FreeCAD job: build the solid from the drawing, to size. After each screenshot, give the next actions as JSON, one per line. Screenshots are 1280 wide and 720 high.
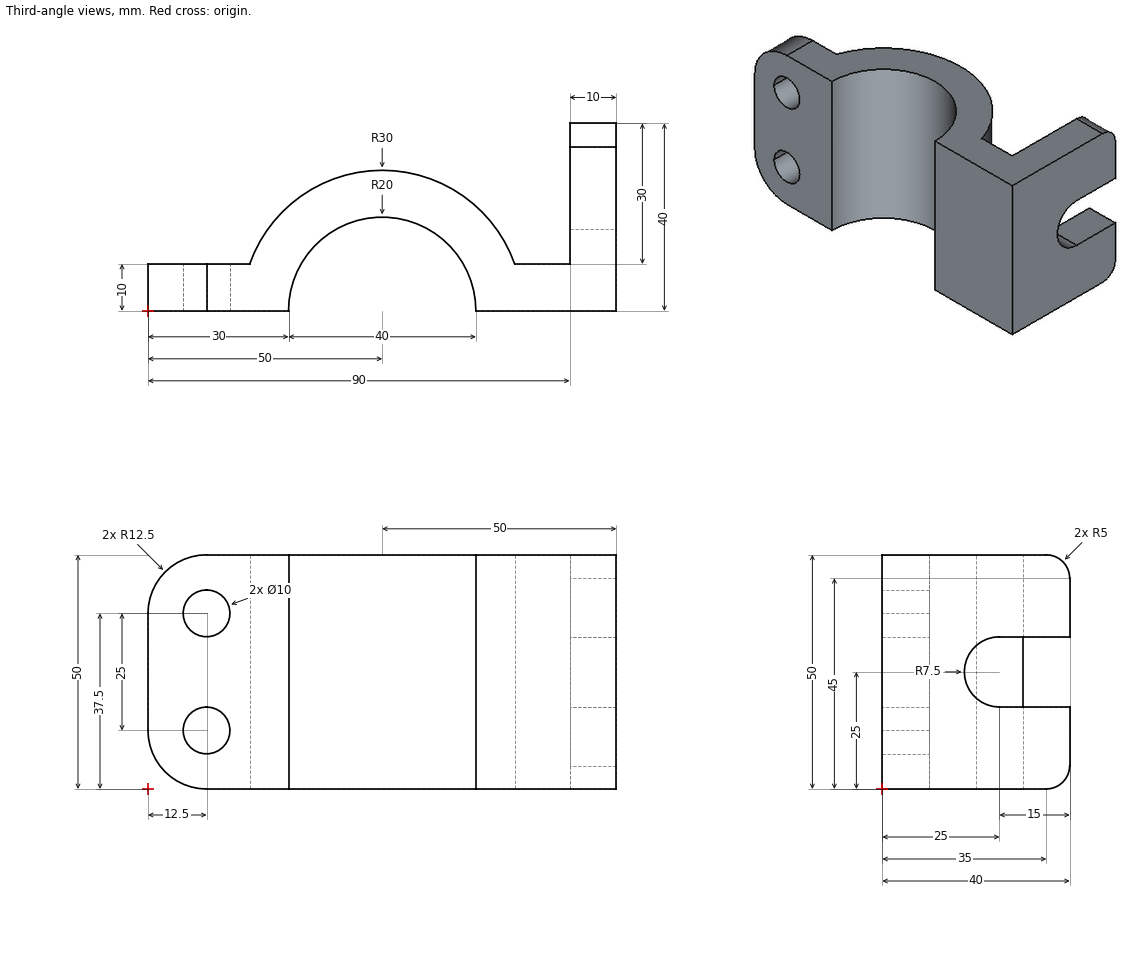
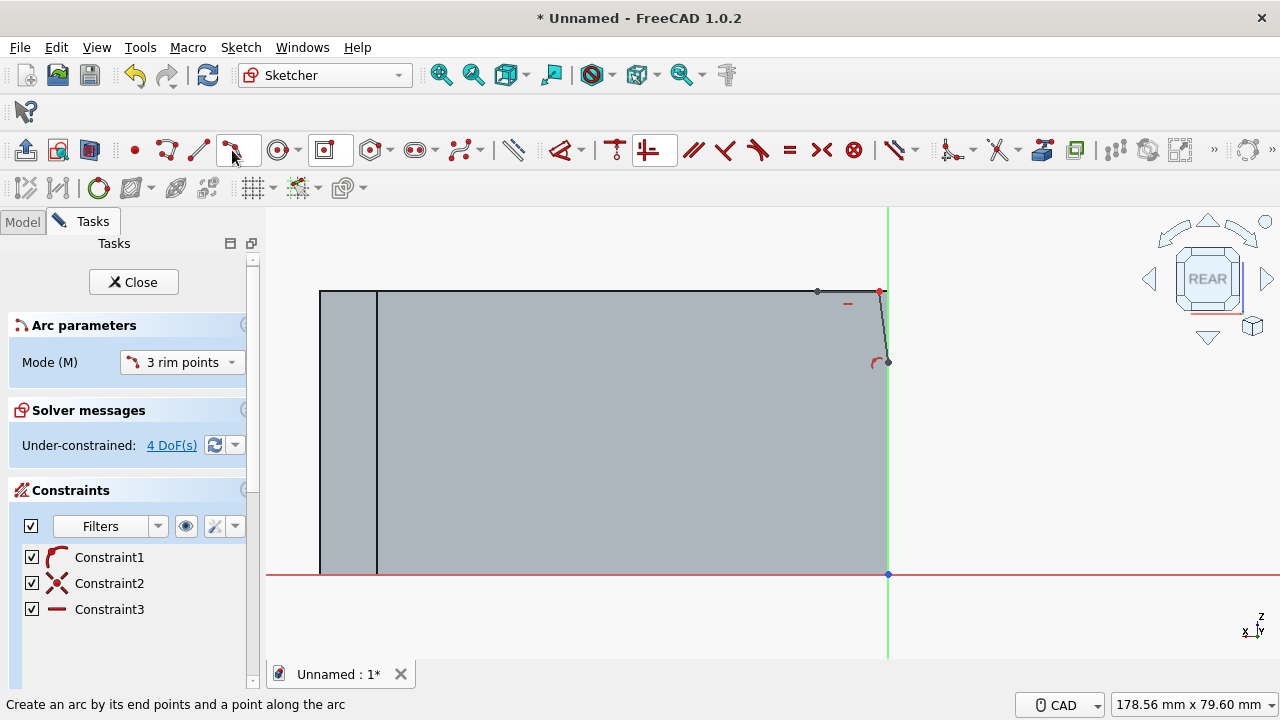
{"action": "left_click", "coordinate": [817, 292]}
{"action": "left_click", "coordinate": [888, 363]}
{"action": "left_click", "coordinate": [868, 312]}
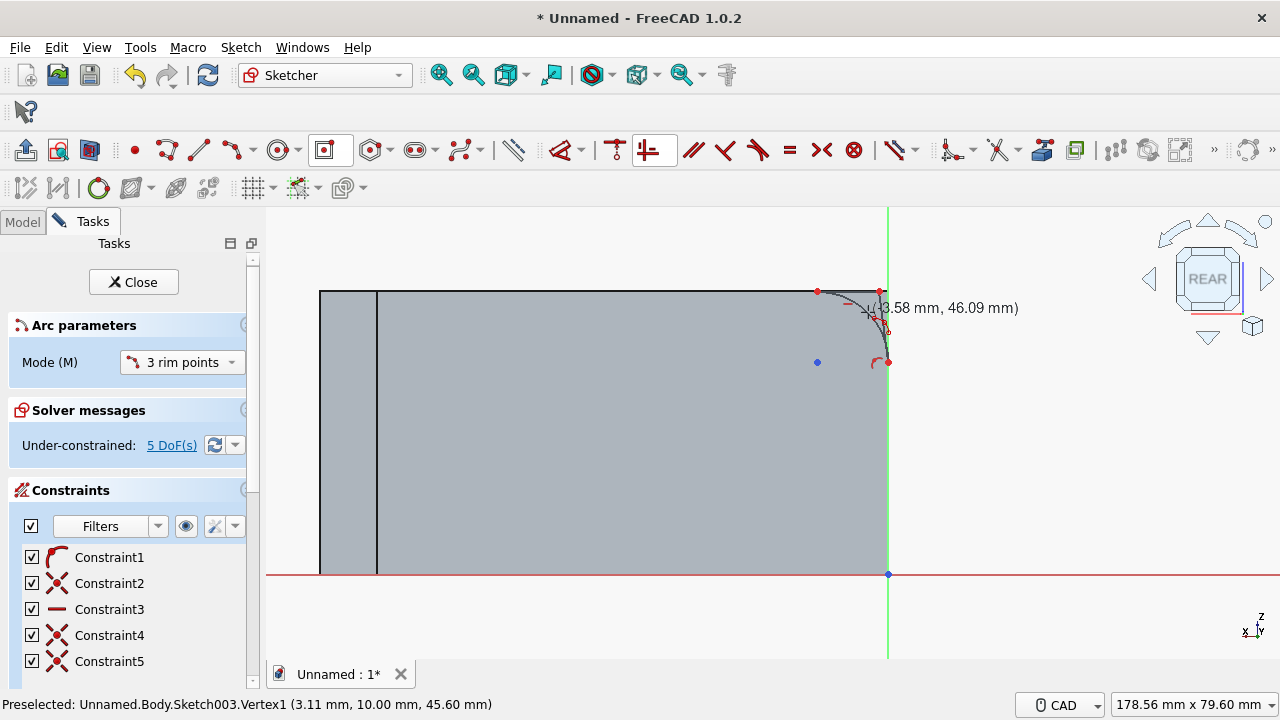
{"action": "left_click", "coordinate": [168, 150]}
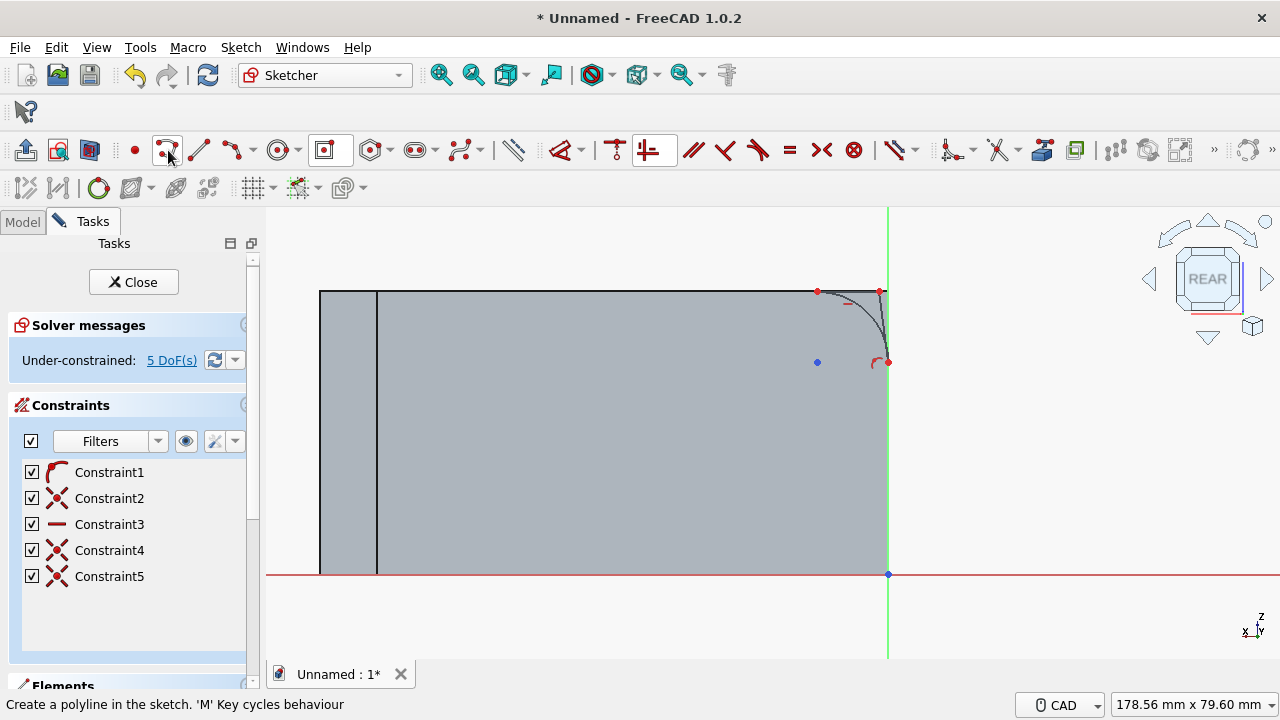
{"action": "left_click", "coordinate": [817, 575]}
{"action": "left_click", "coordinate": [888, 575]}
{"action": "left_click", "coordinate": [879, 504]}
{"action": "right_click", "coordinate": [879, 504]}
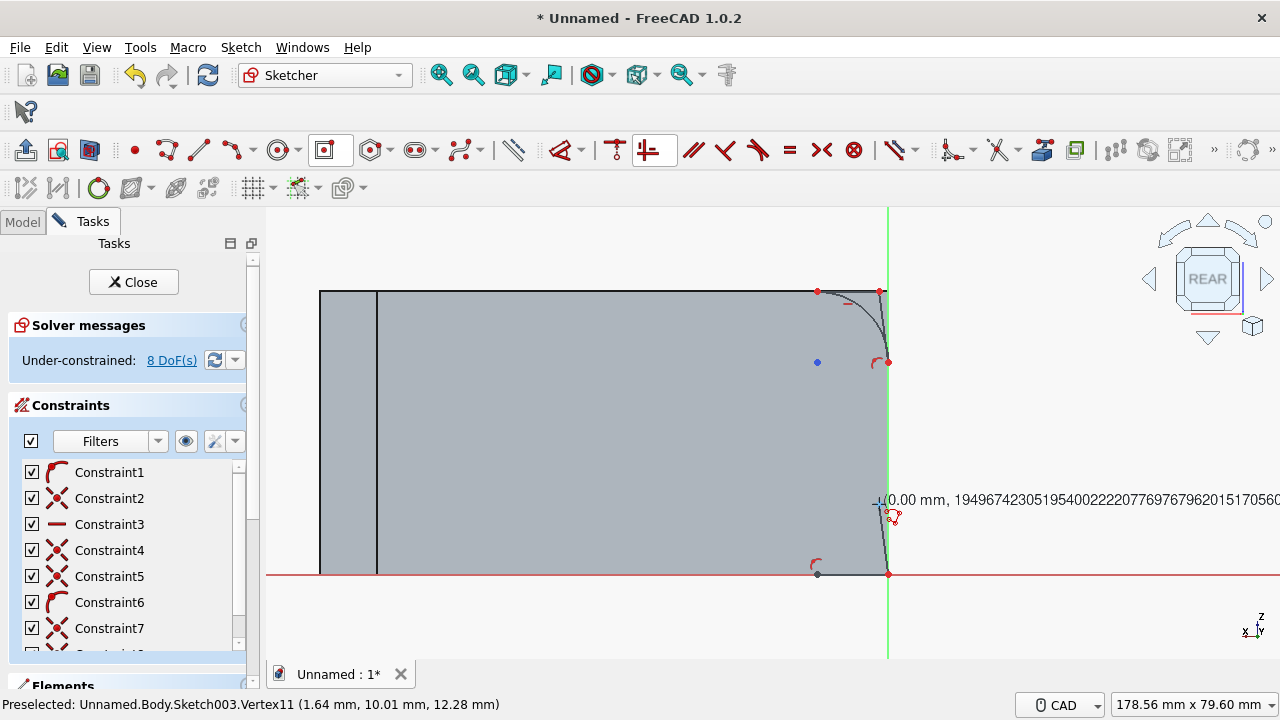
{"action": "left_click", "coordinate": [232, 150]}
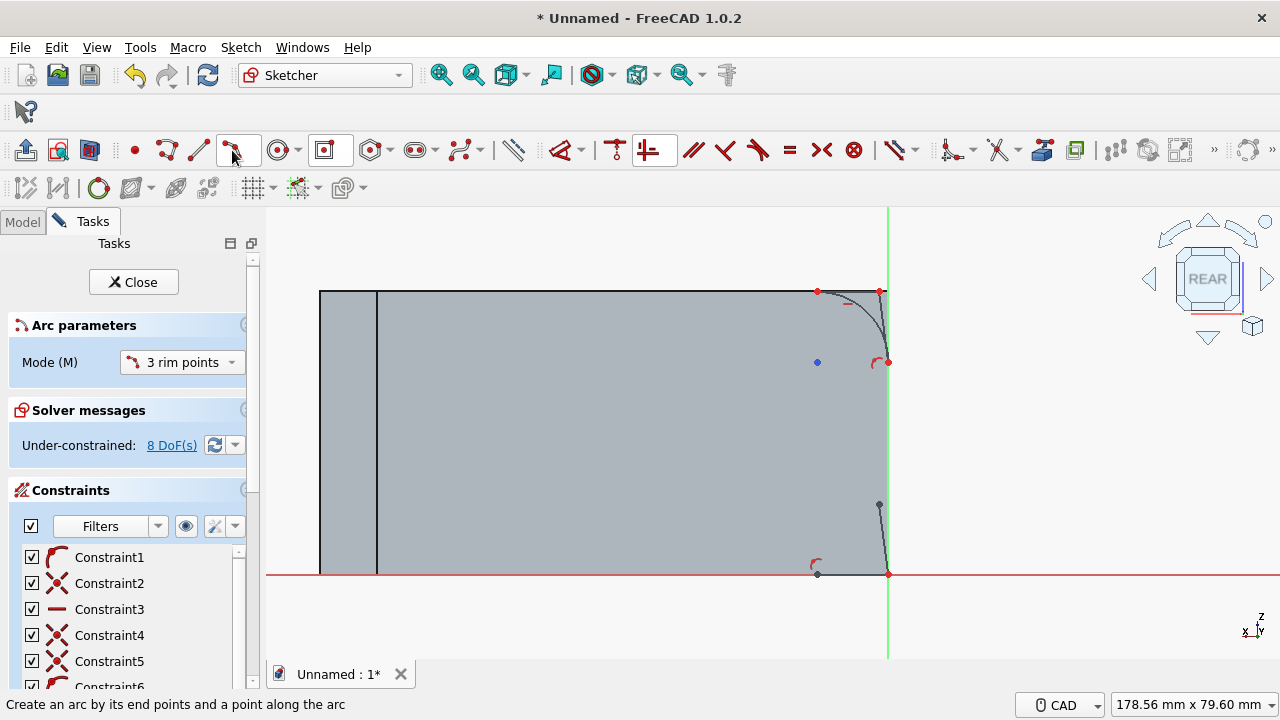
{"action": "left_click", "coordinate": [879, 505]}
{"action": "left_click", "coordinate": [817, 575]}
{"action": "left_click", "coordinate": [868, 554]}
{"action": "key", "text": "Escape"}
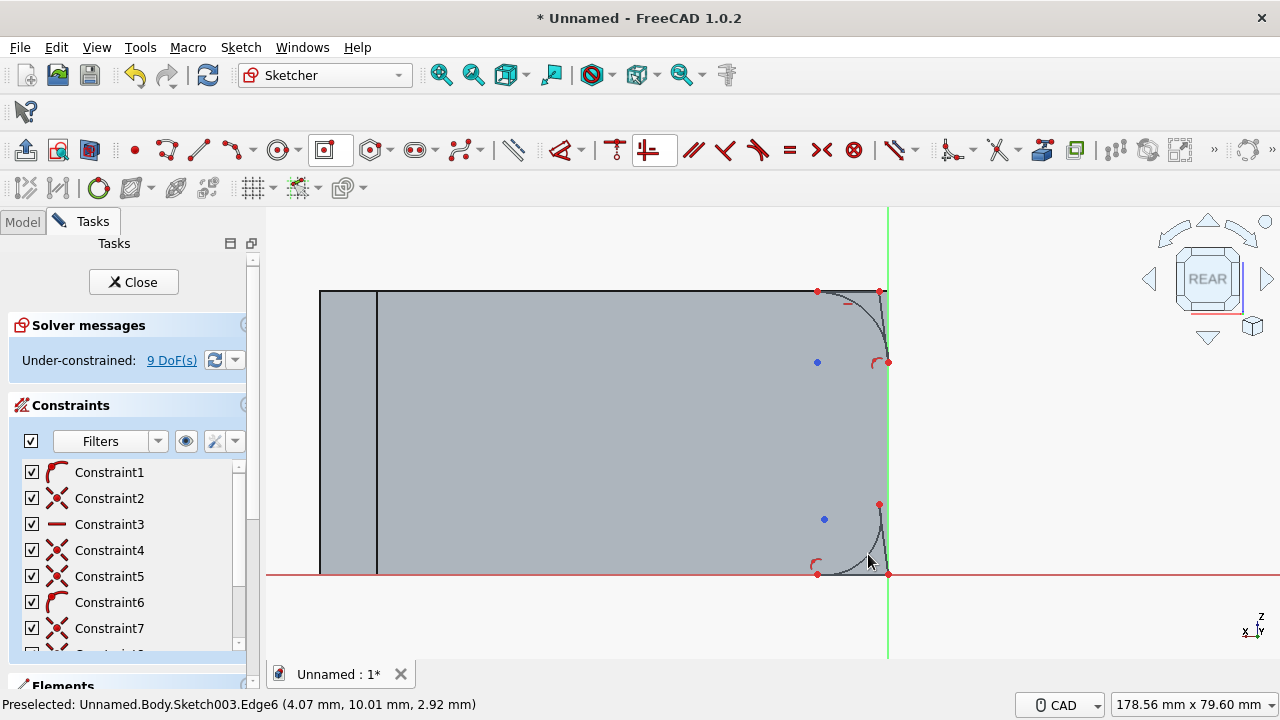
{"action": "scroll", "coordinate": [881, 306], "scroll_direction": "up", "scroll_amount": 4}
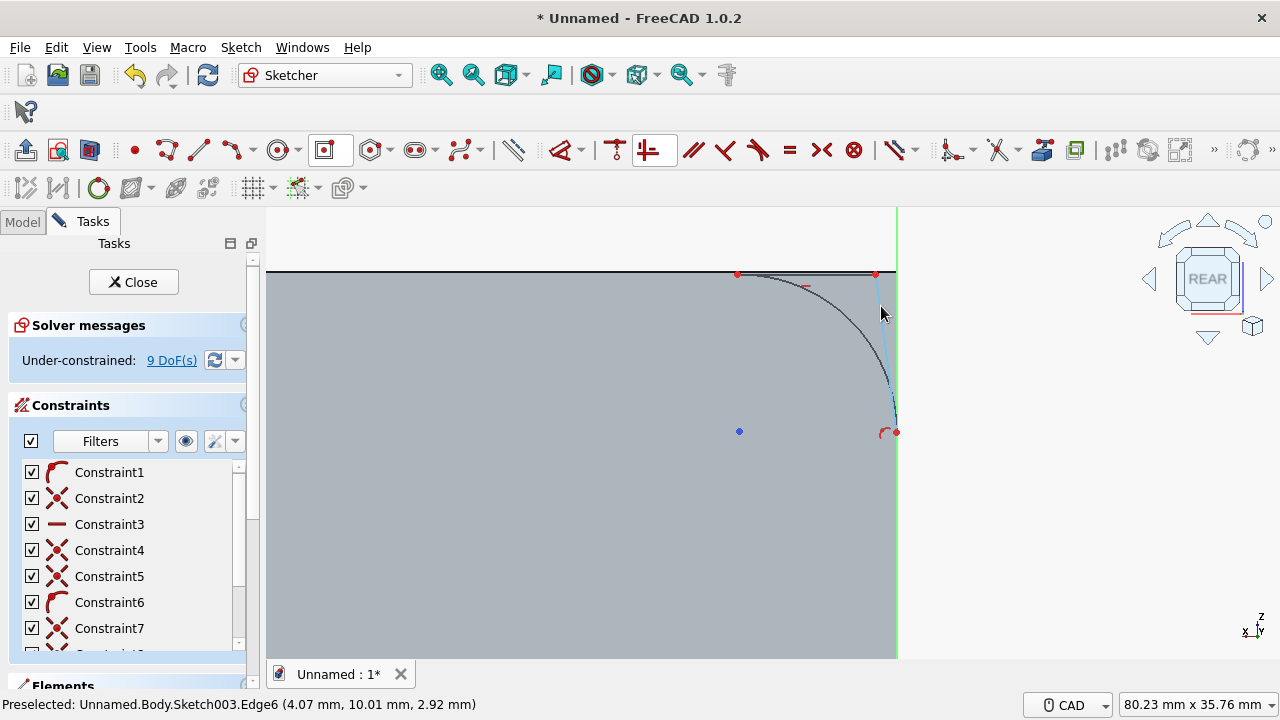
{"action": "left_click", "coordinate": [880, 306]}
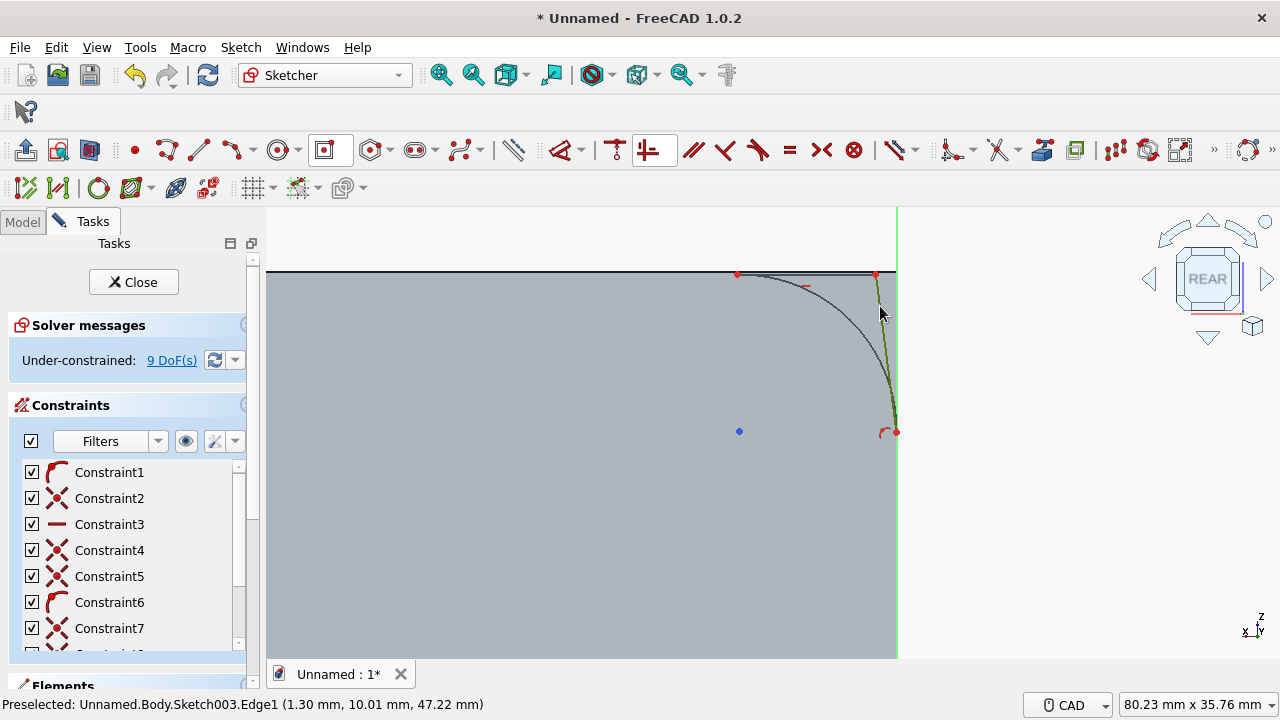
{"action": "left_click", "coordinate": [810, 291]}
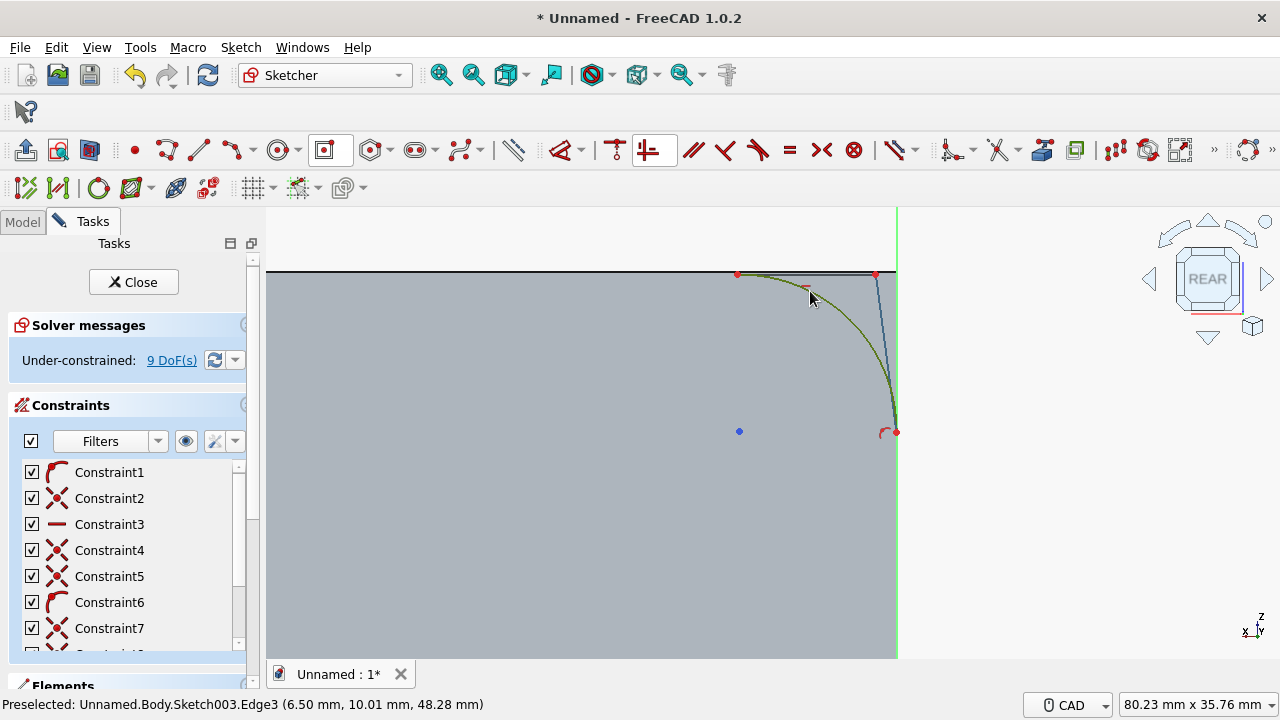
{"action": "left_click", "coordinate": [758, 150]}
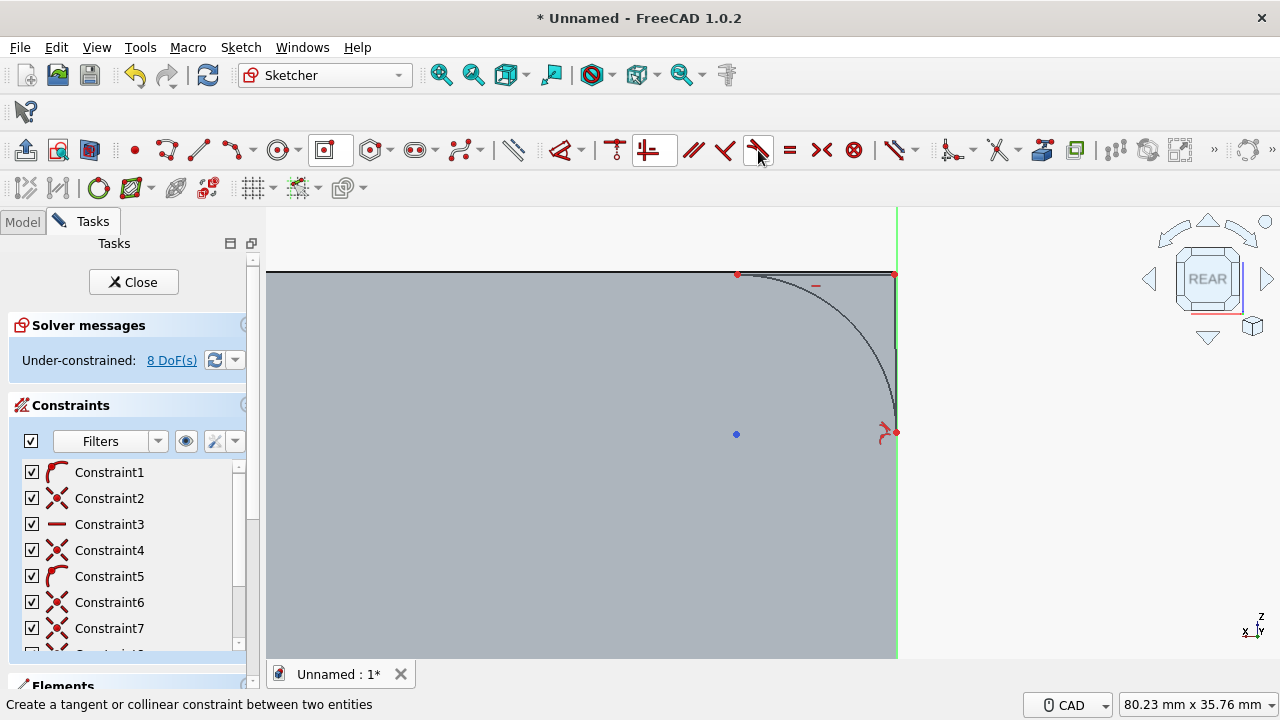
{"action": "left_click", "coordinate": [848, 275]}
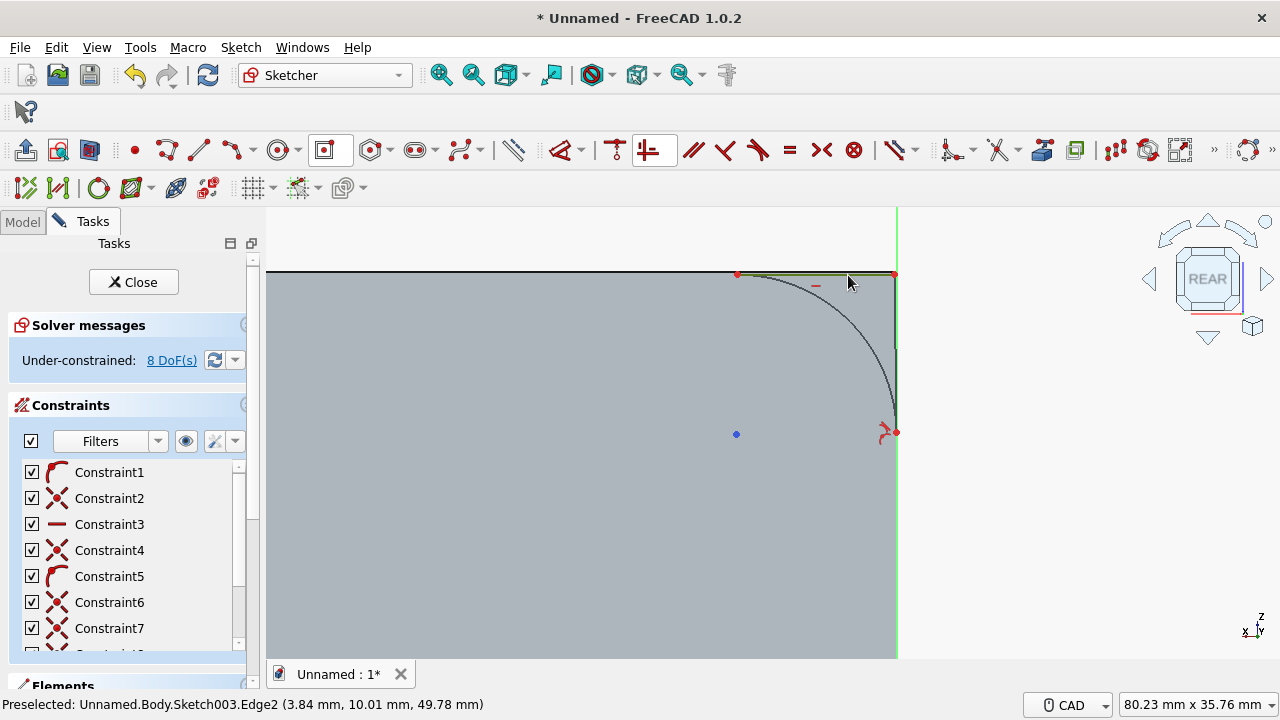
{"action": "left_click", "coordinate": [879, 361]}